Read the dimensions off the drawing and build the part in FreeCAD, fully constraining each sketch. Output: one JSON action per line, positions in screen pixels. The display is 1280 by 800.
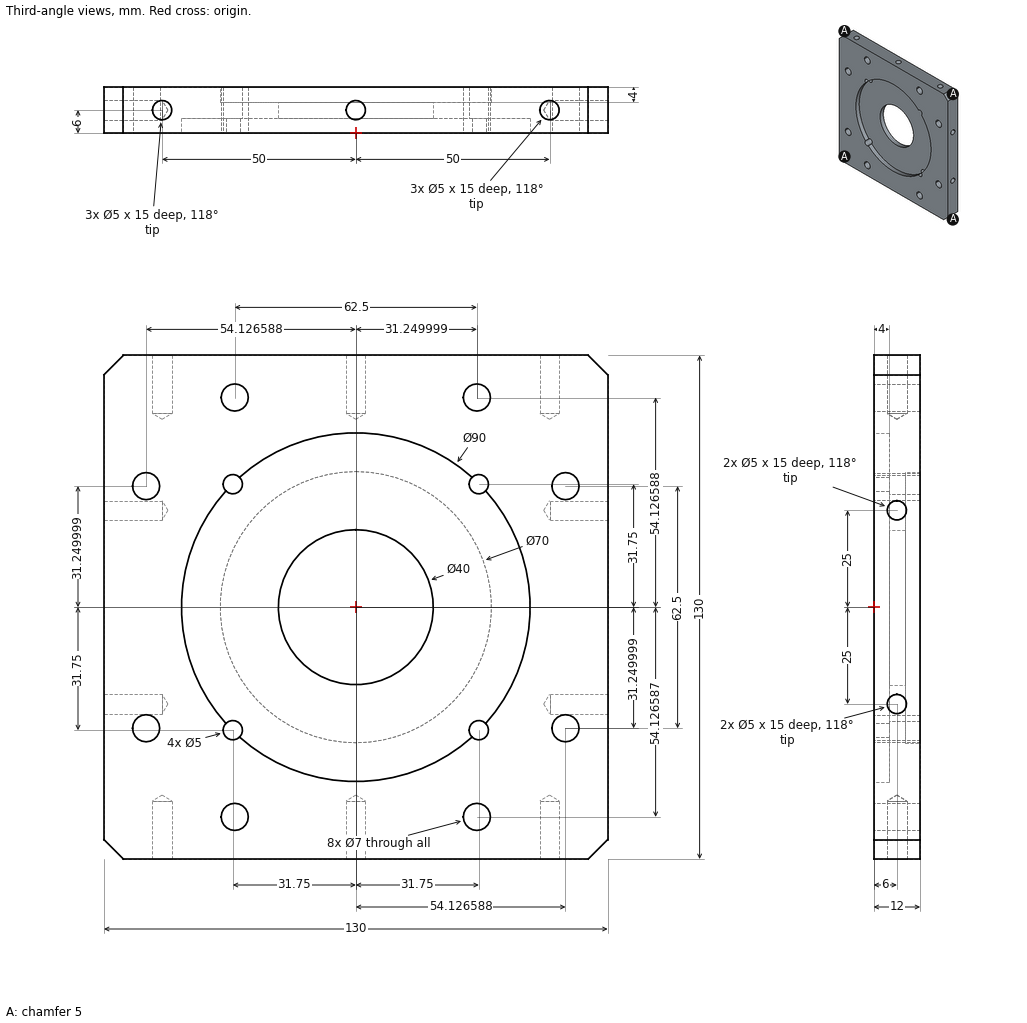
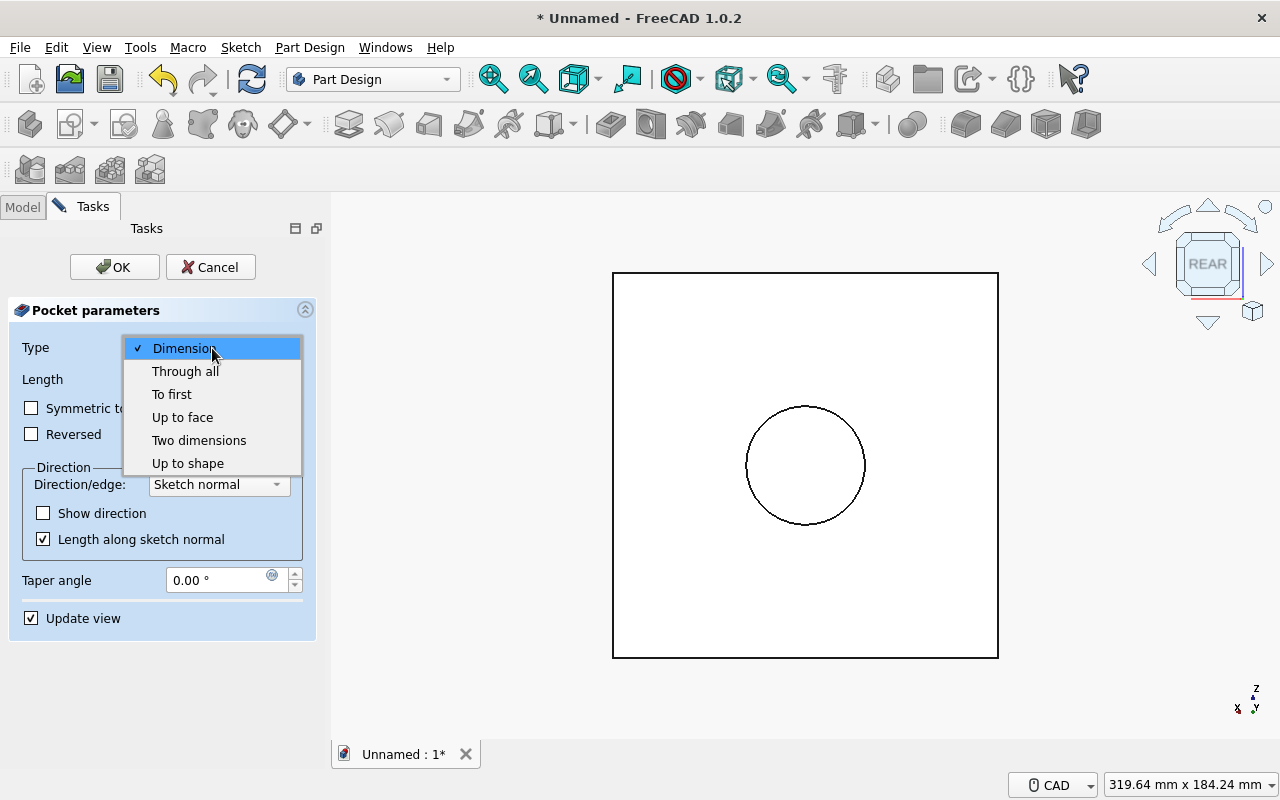
{"action": "left_click", "coordinate": [212, 372]}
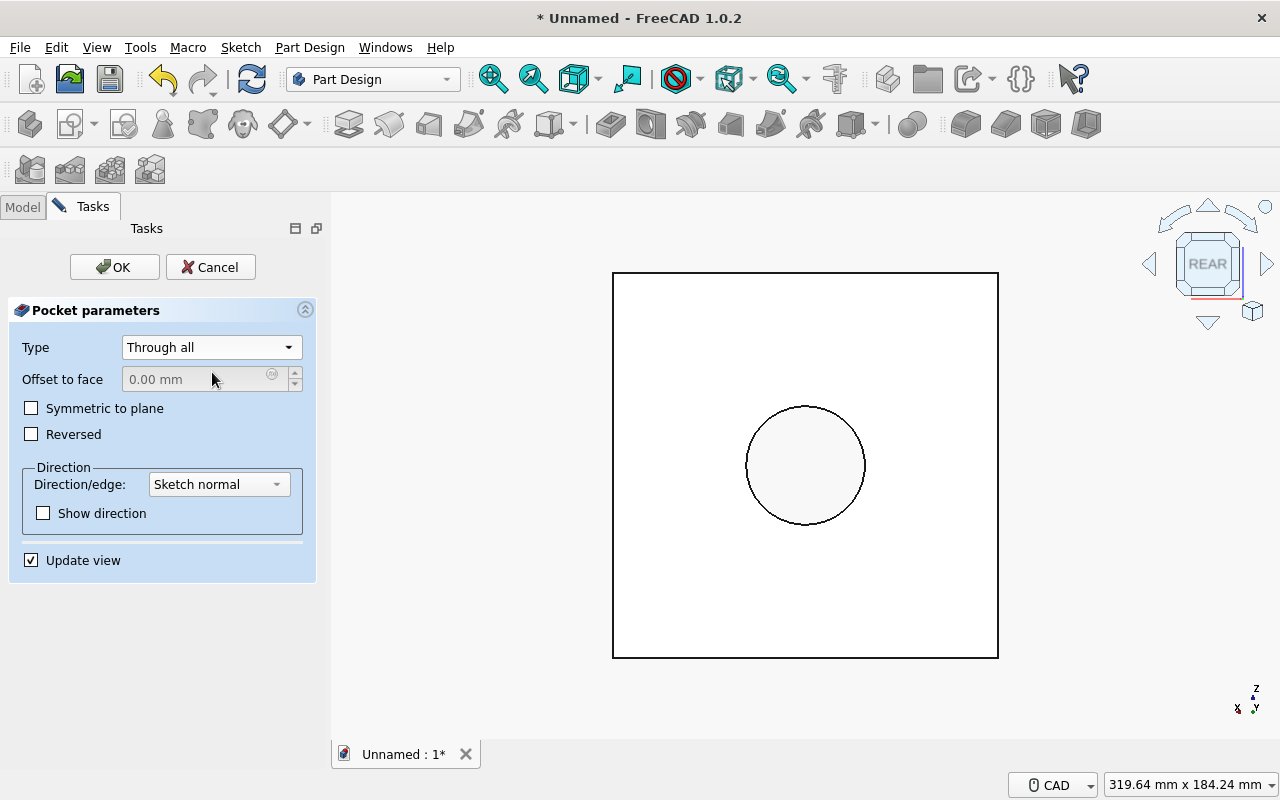
{"action": "left_click", "coordinate": [115, 267]}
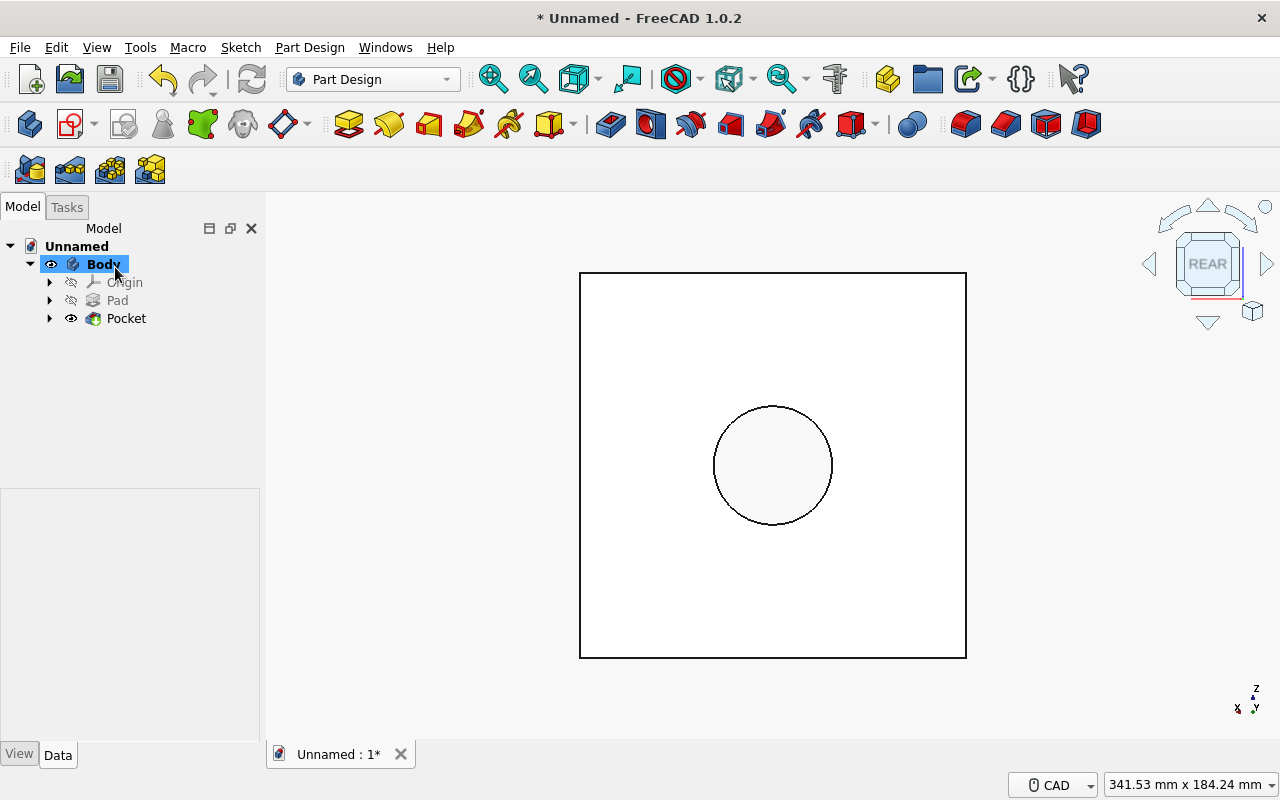
{"action": "left_click", "coordinate": [663, 354]}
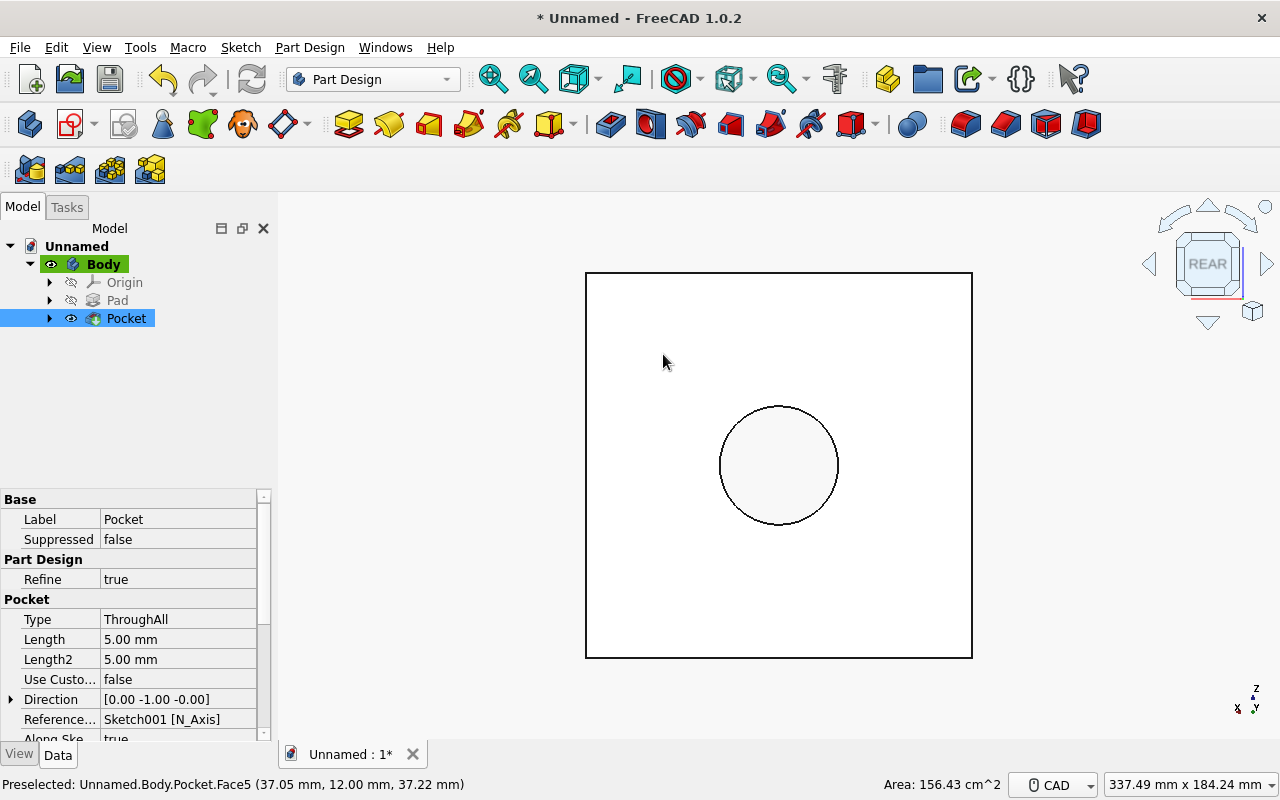
{"action": "left_click", "coordinate": [70, 124]}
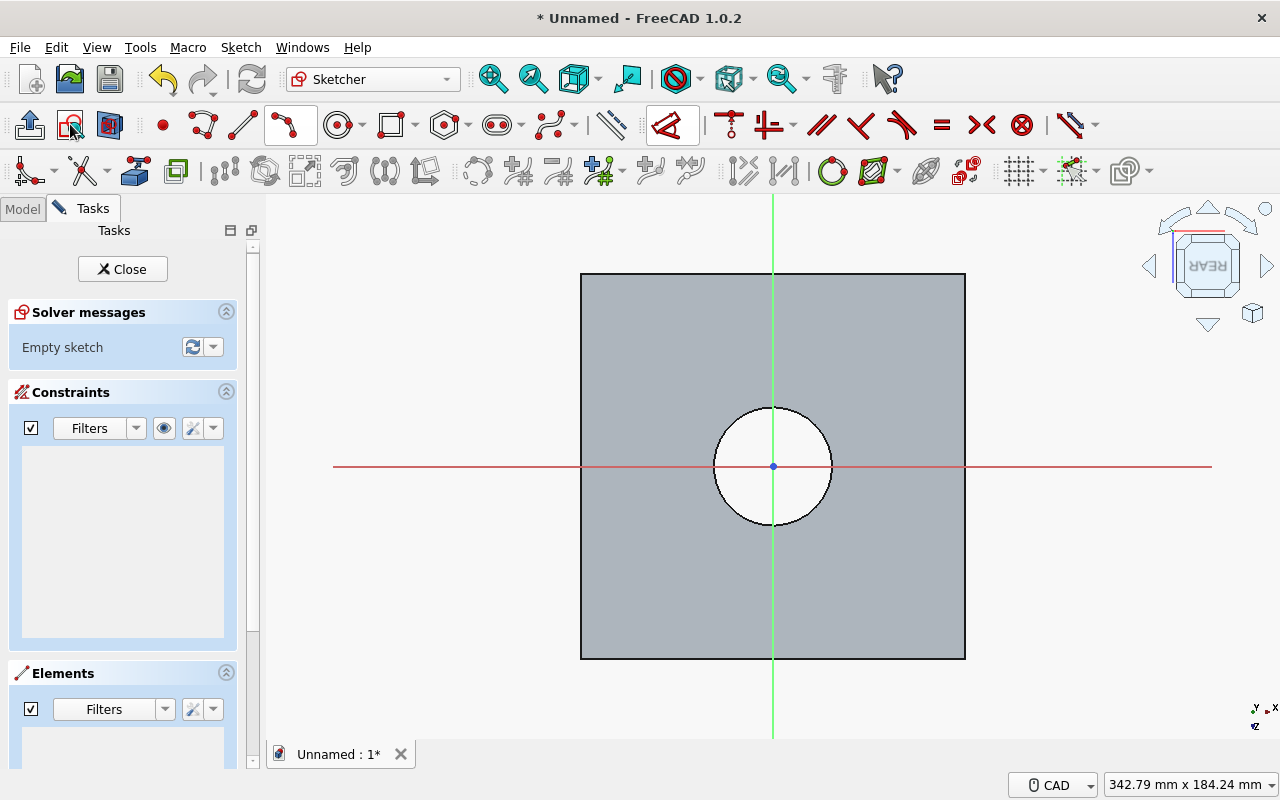
{"action": "key", "text": "g c"}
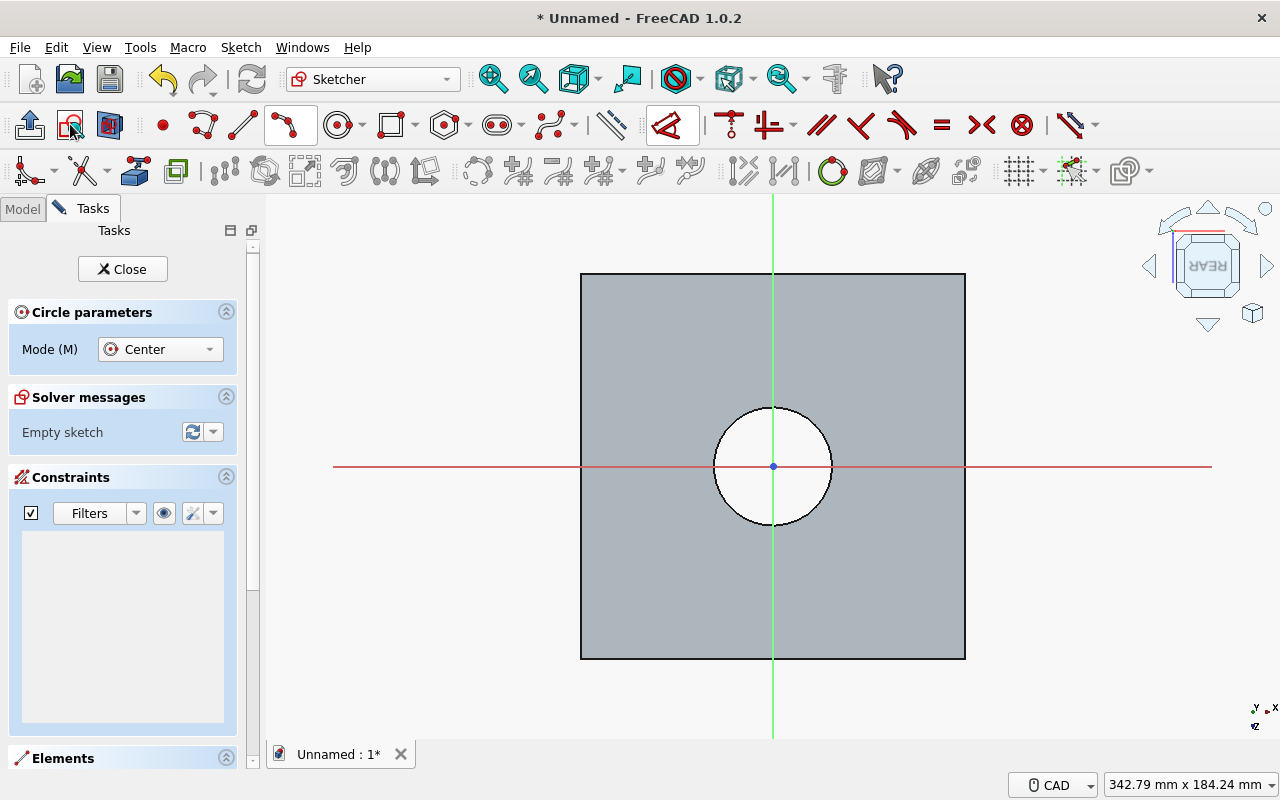
{"action": "scroll", "coordinate": [865, 306], "scroll_direction": "up", "scroll_amount": 4}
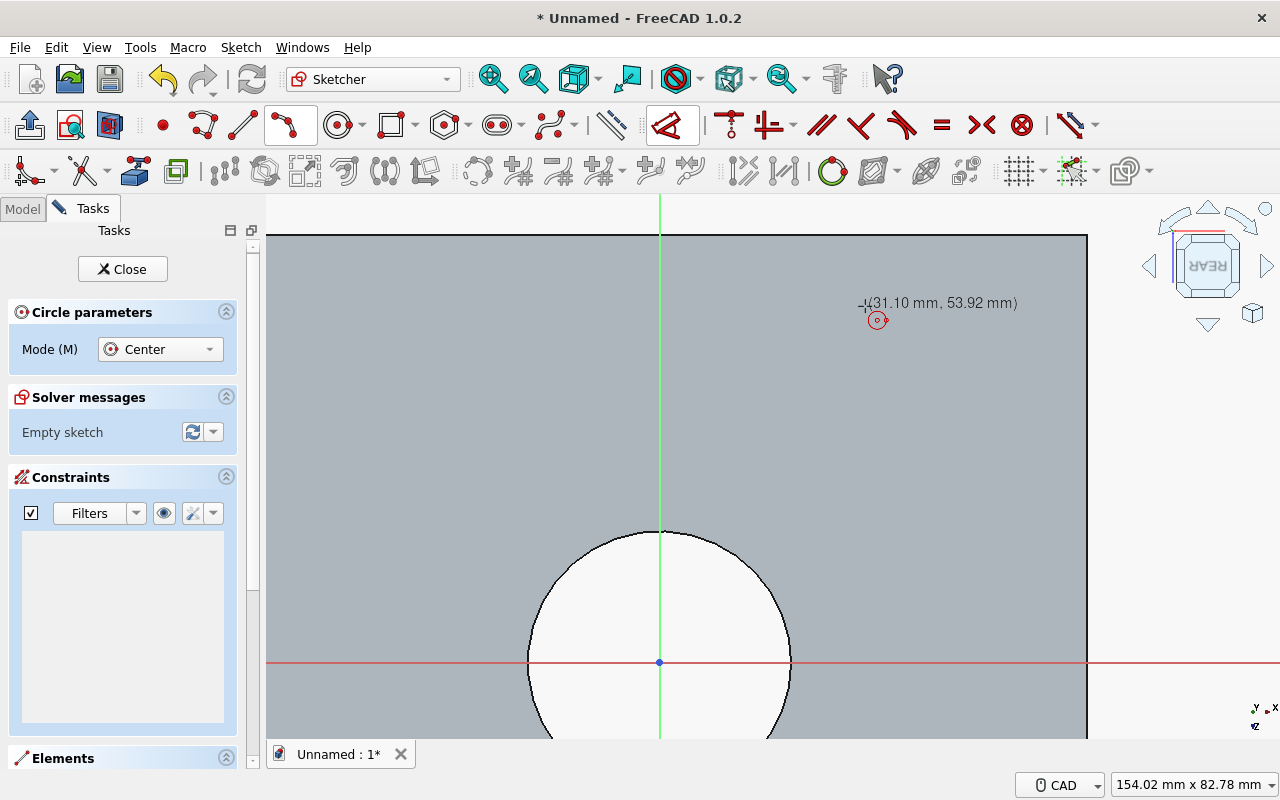
{"action": "left_click", "coordinate": [865, 307]}
{"action": "left_click", "coordinate": [882, 290]}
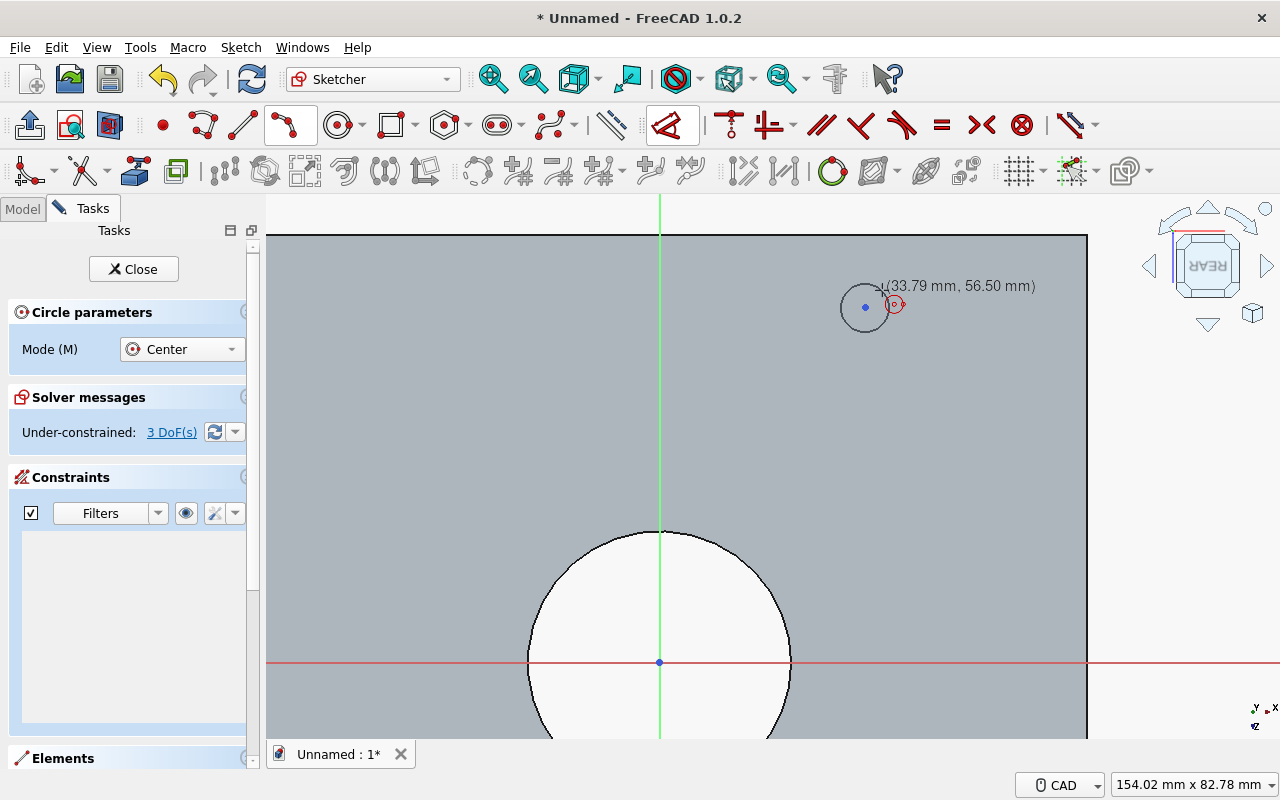
{"action": "left_click", "coordinate": [1016, 457]}
{"action": "left_click", "coordinate": [1032, 441]}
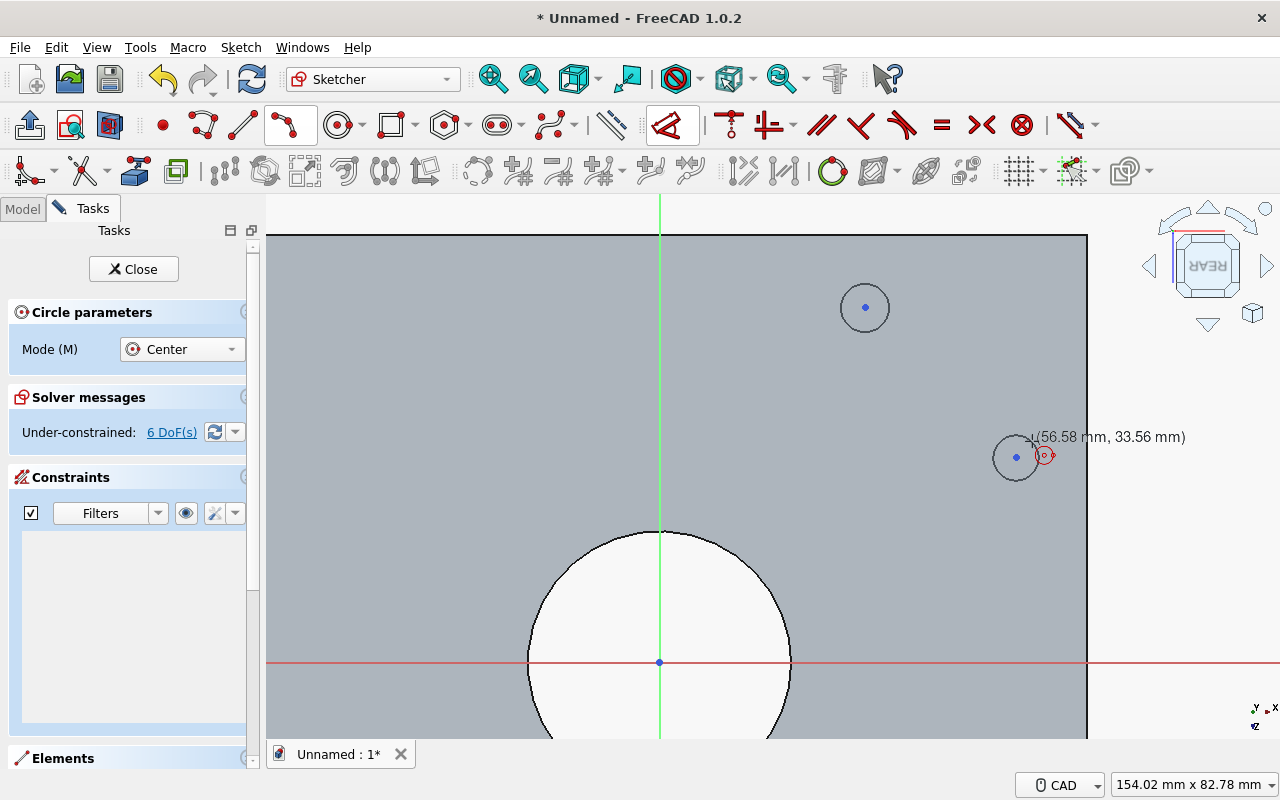
{"action": "scroll", "coordinate": [741, 306], "scroll_direction": "down", "scroll_amount": 4}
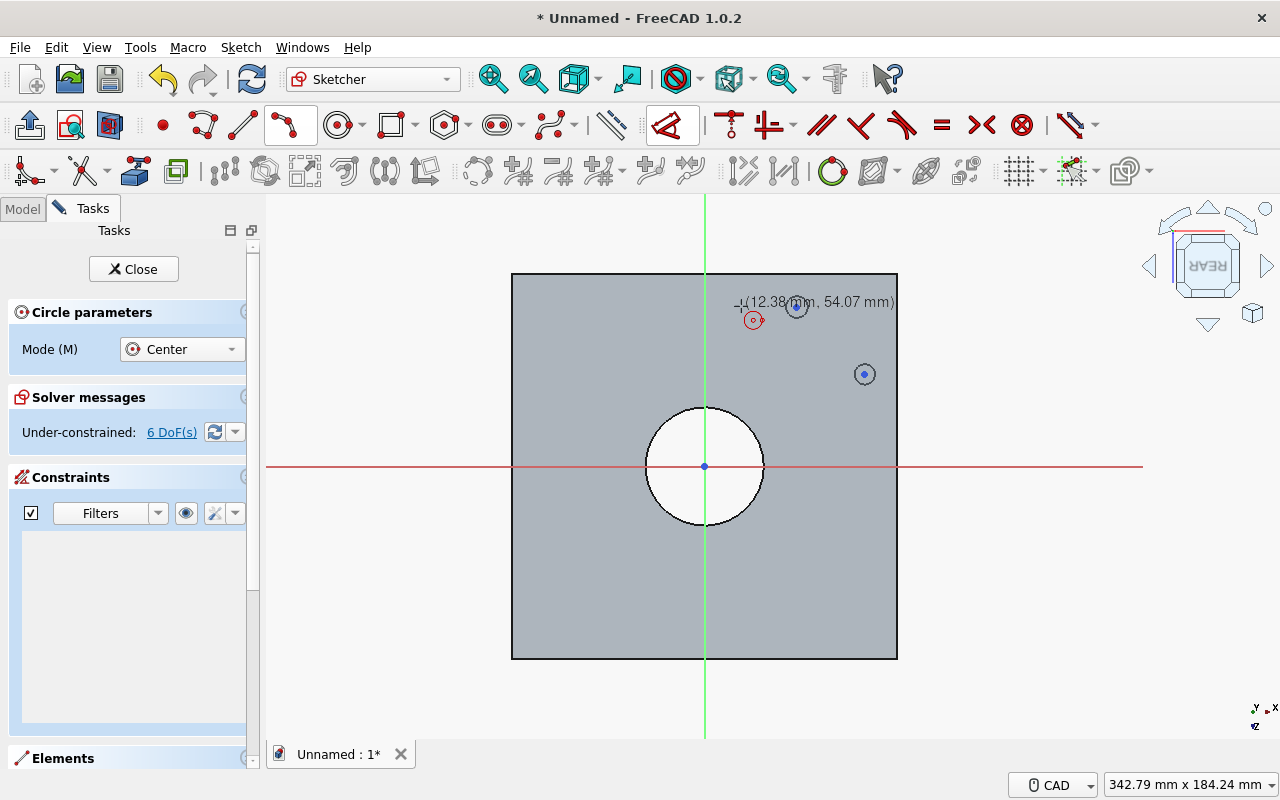
{"action": "scroll", "coordinate": [865, 559], "scroll_direction": "up", "scroll_amount": 4}